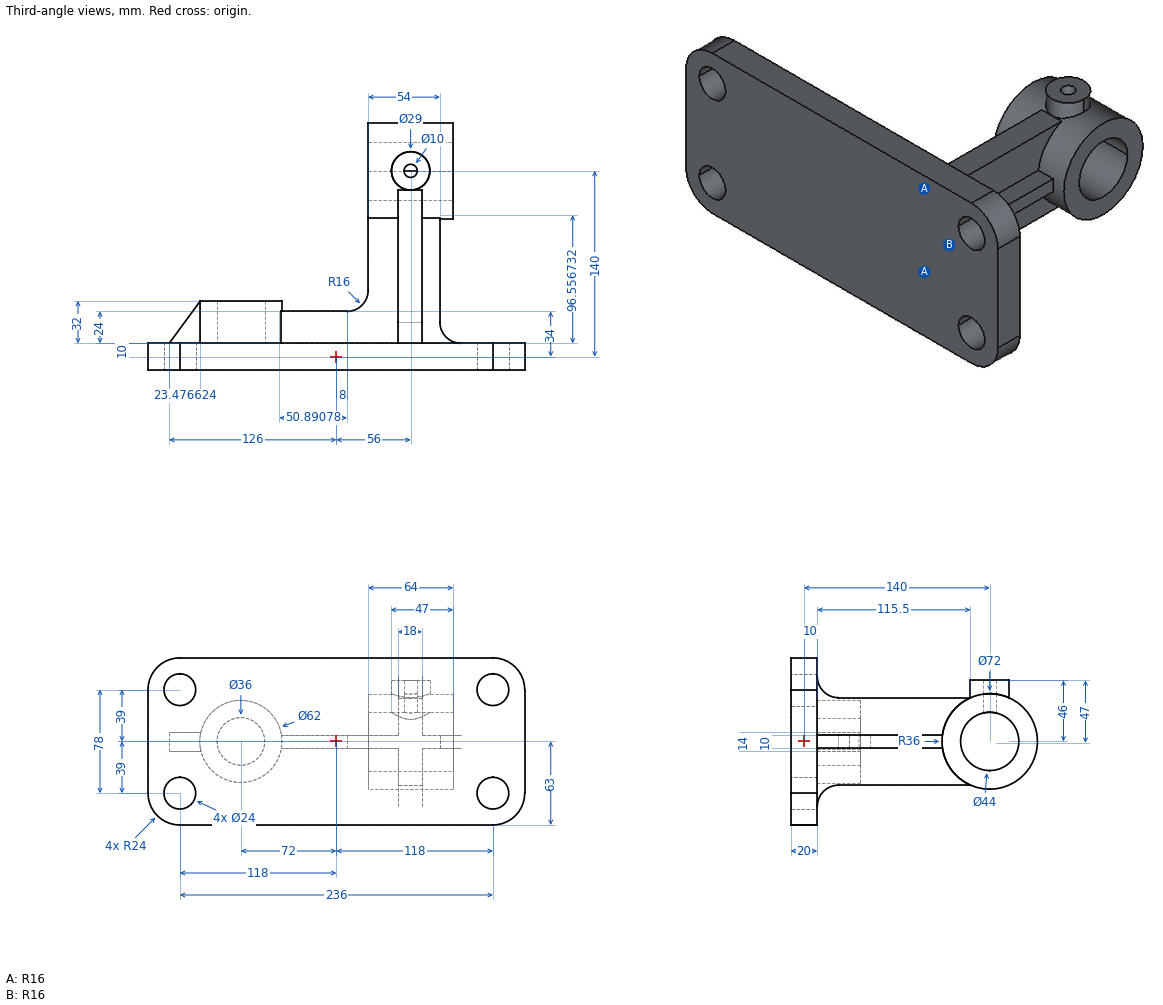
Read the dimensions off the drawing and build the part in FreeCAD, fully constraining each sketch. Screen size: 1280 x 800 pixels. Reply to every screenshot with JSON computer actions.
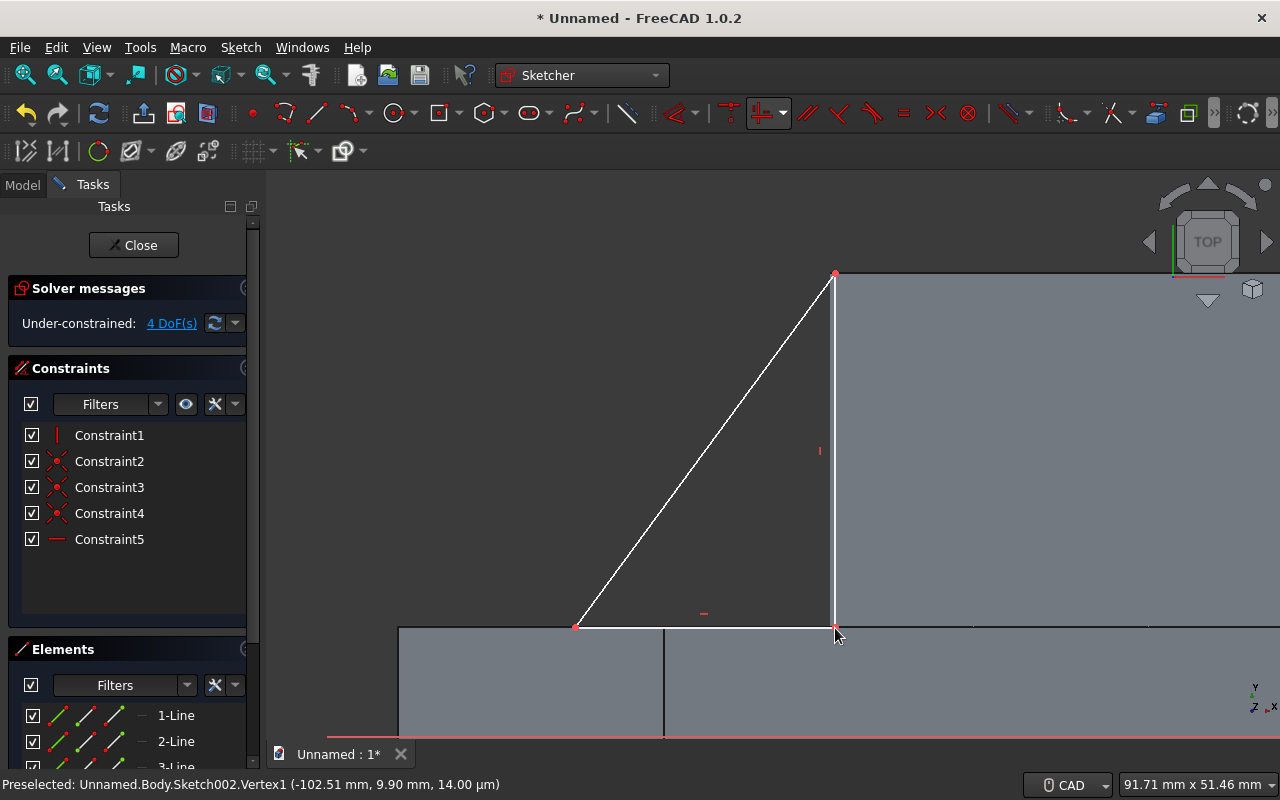
{"action": "left_click", "coordinate": [674, 114]}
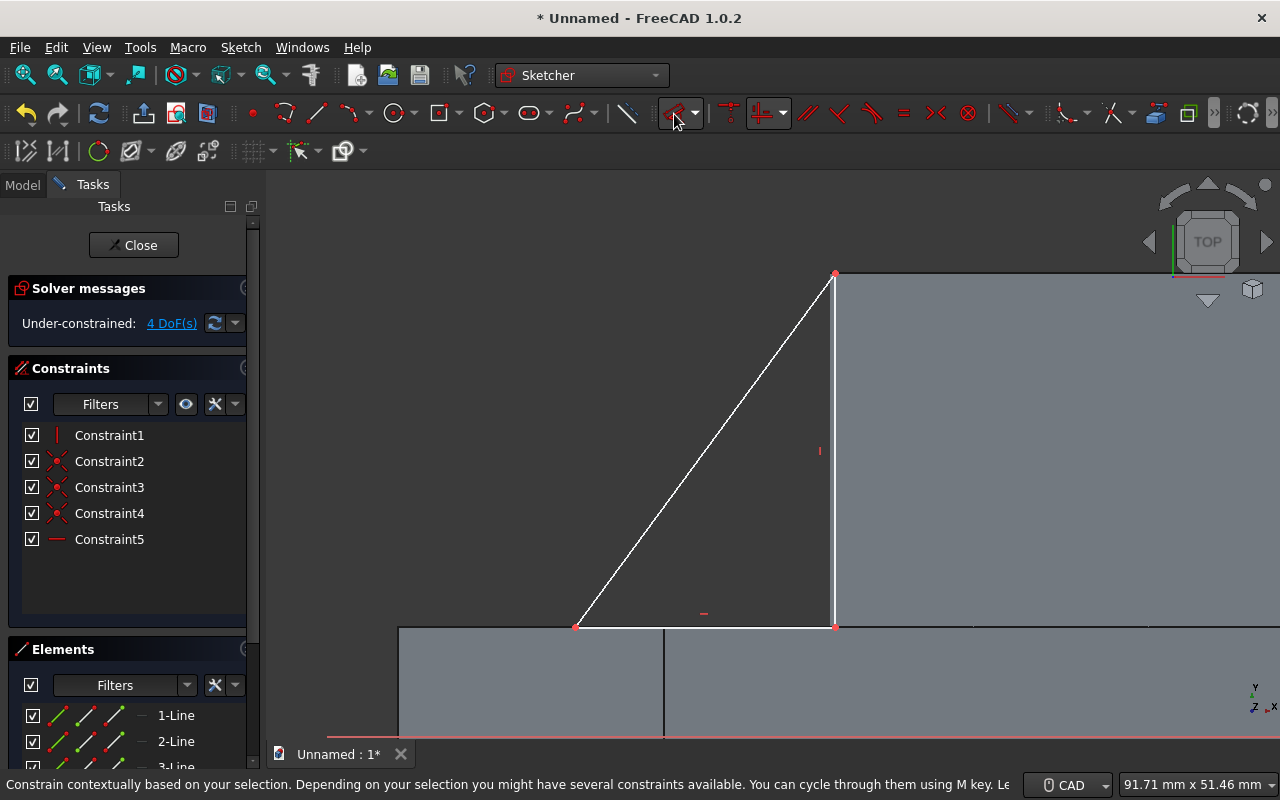
{"action": "left_click", "coordinate": [835, 522]}
{"action": "left_click", "coordinate": [869, 451]}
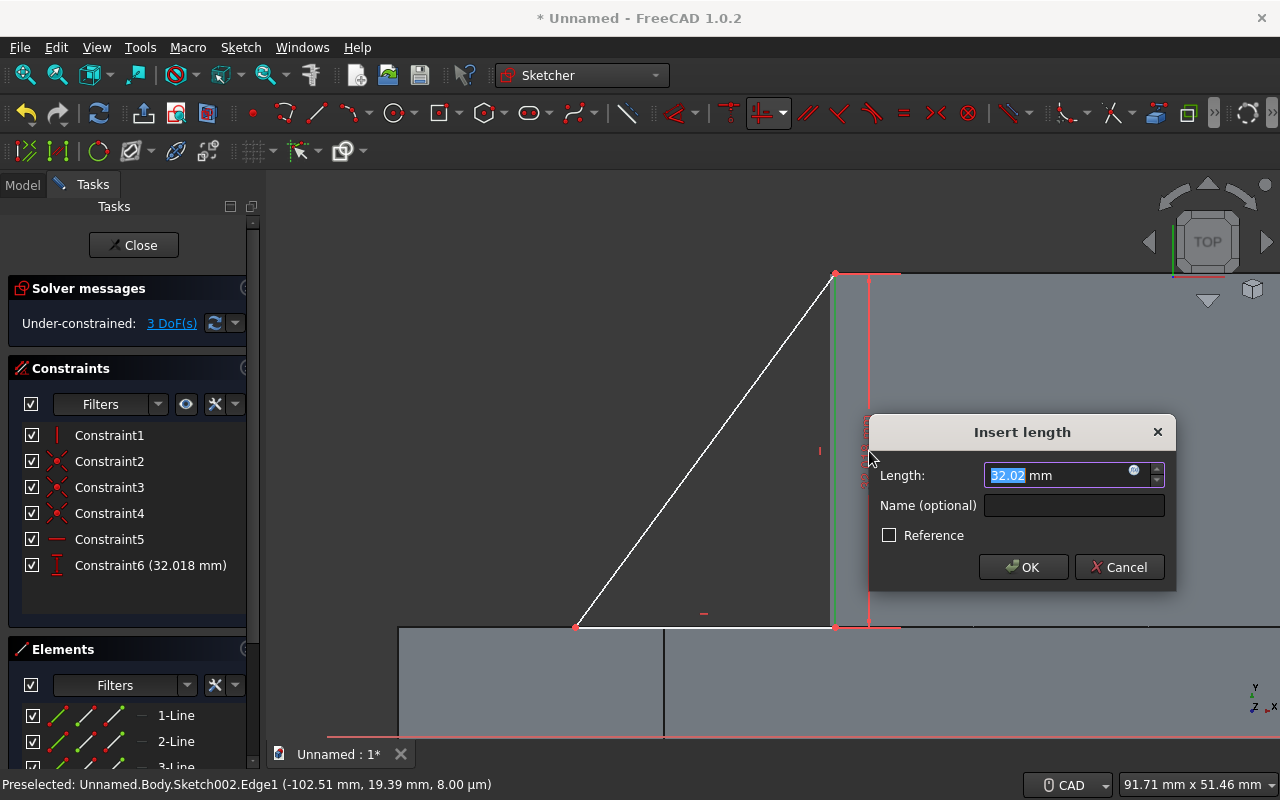
{"action": "type", "text": "32"}
{"action": "key", "text": "Return"}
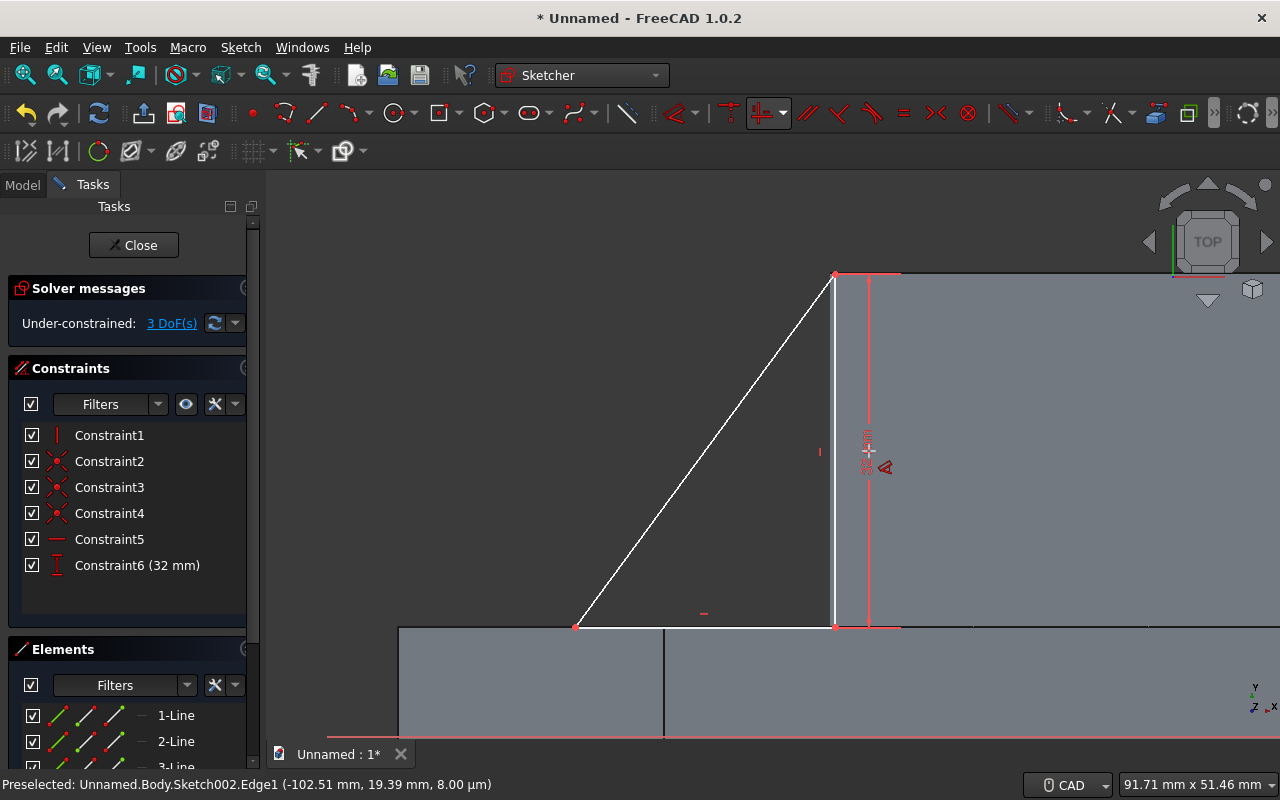
{"action": "left_click", "coordinate": [835, 628]}
{"action": "left_click", "coordinate": [801, 669]}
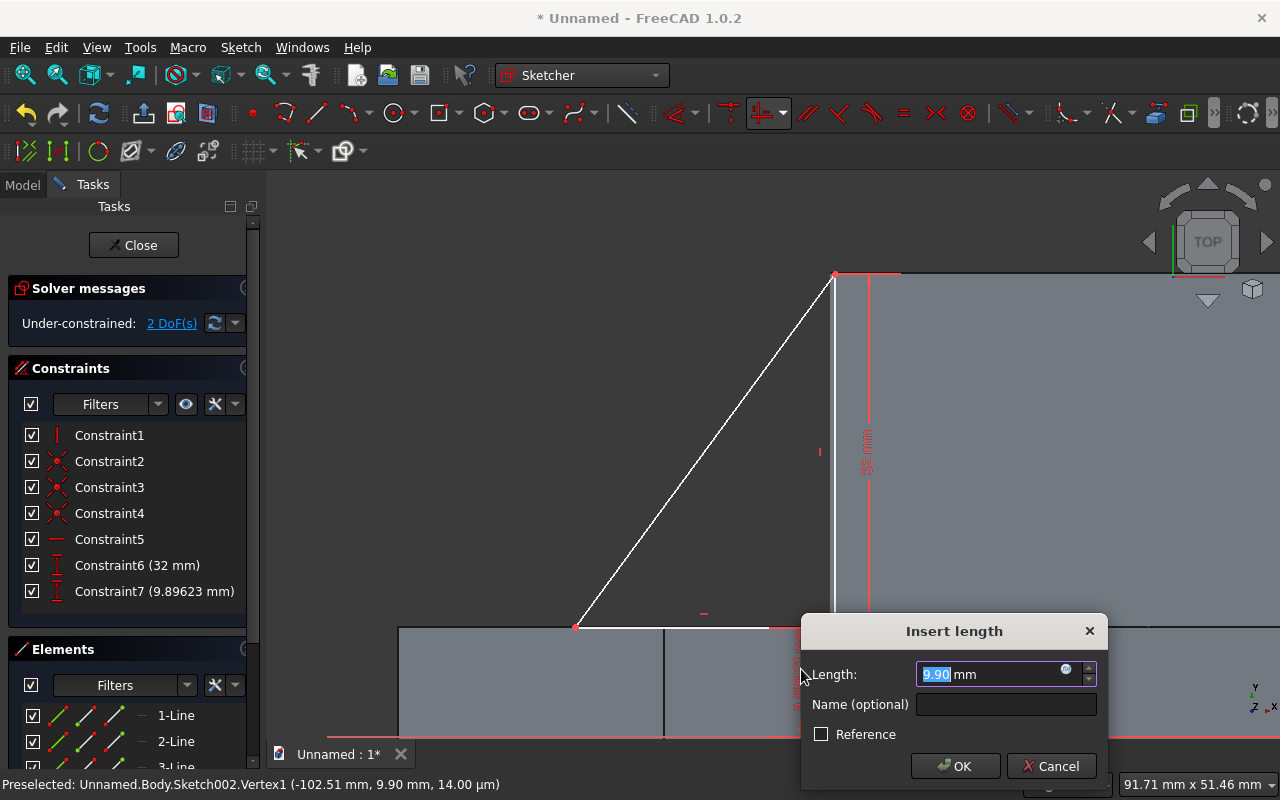
{"action": "type", "text": "10"}
{"action": "key", "text": "Return"}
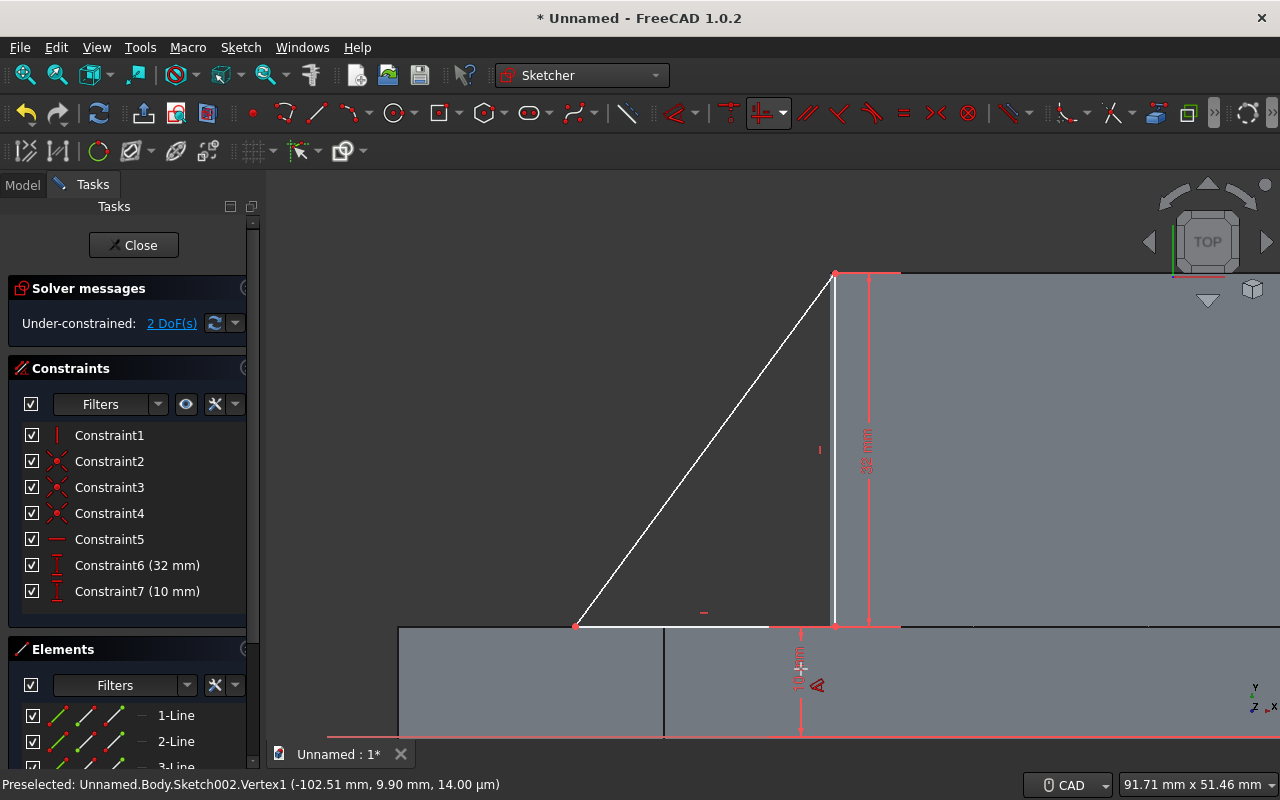
{"action": "left_click", "coordinate": [575, 627]}
{"action": "left_click", "coordinate": [721, 593]}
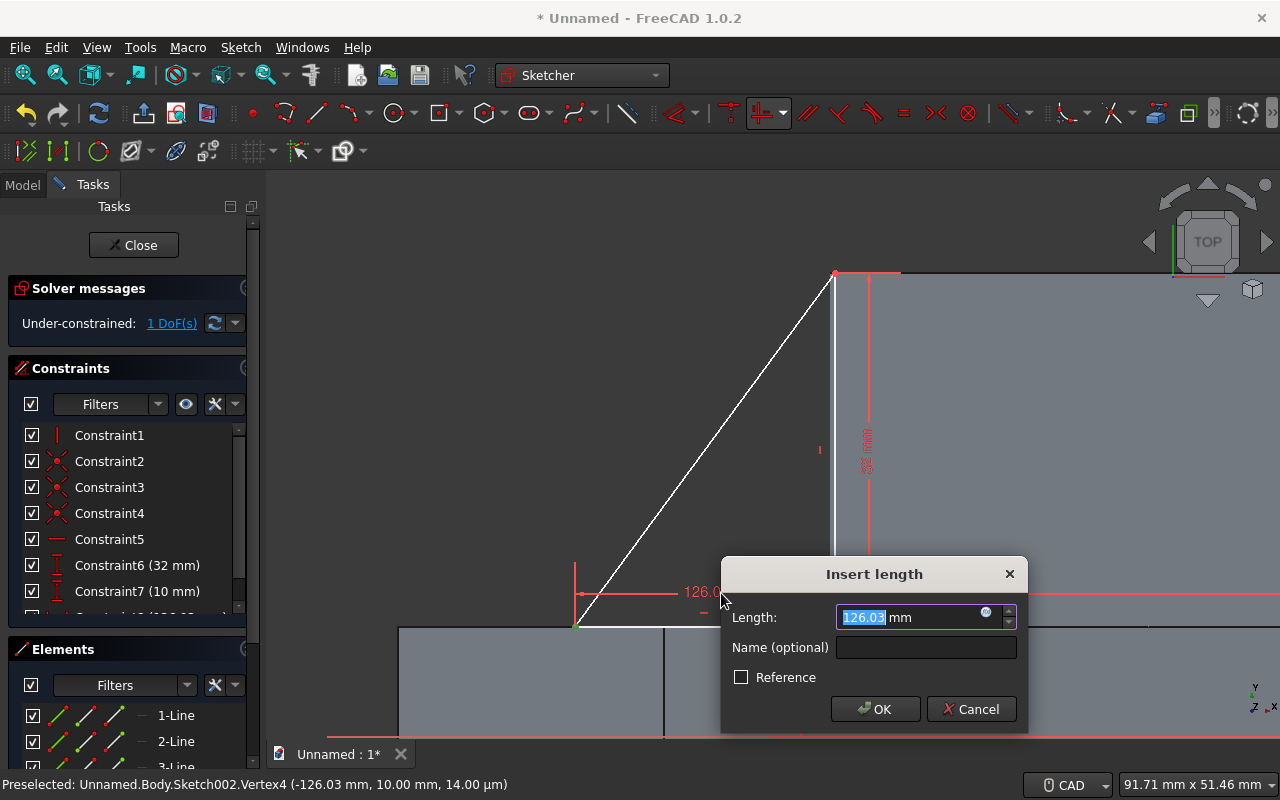
{"action": "type", "text": "126"}
{"action": "key", "text": "Return"}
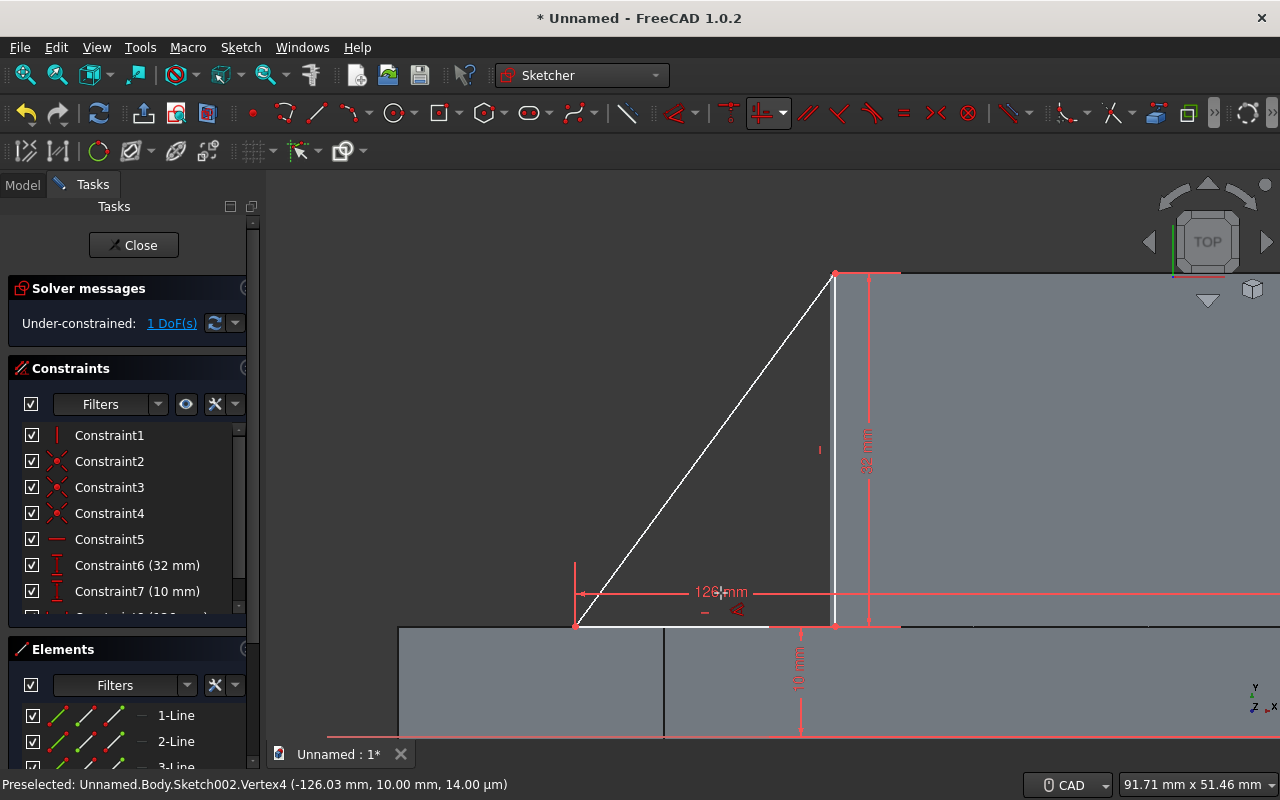
{"action": "left_click", "coordinate": [653, 627]}
{"action": "left_click", "coordinate": [705, 661]}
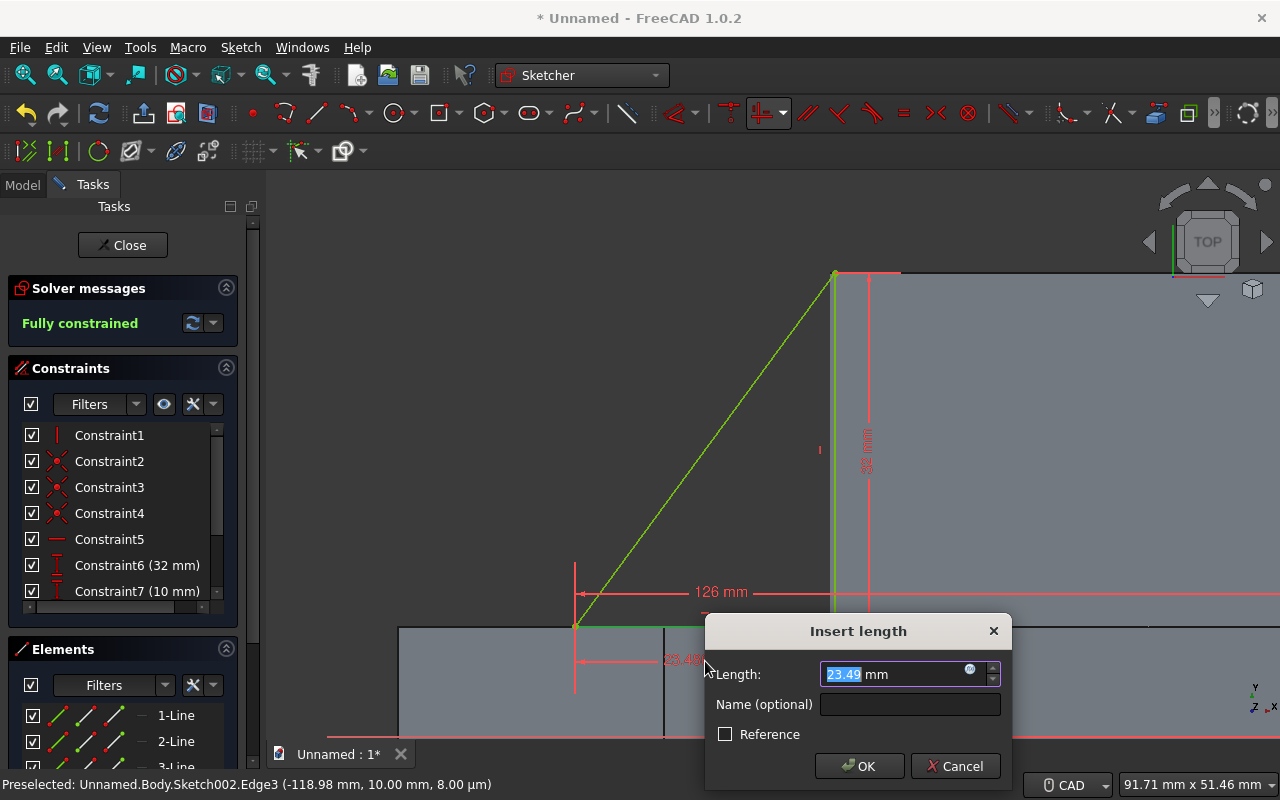
{"action": "type", "text": "23.476624"}
{"action": "key", "text": "Return"}
{"action": "key", "text": "Escape"}